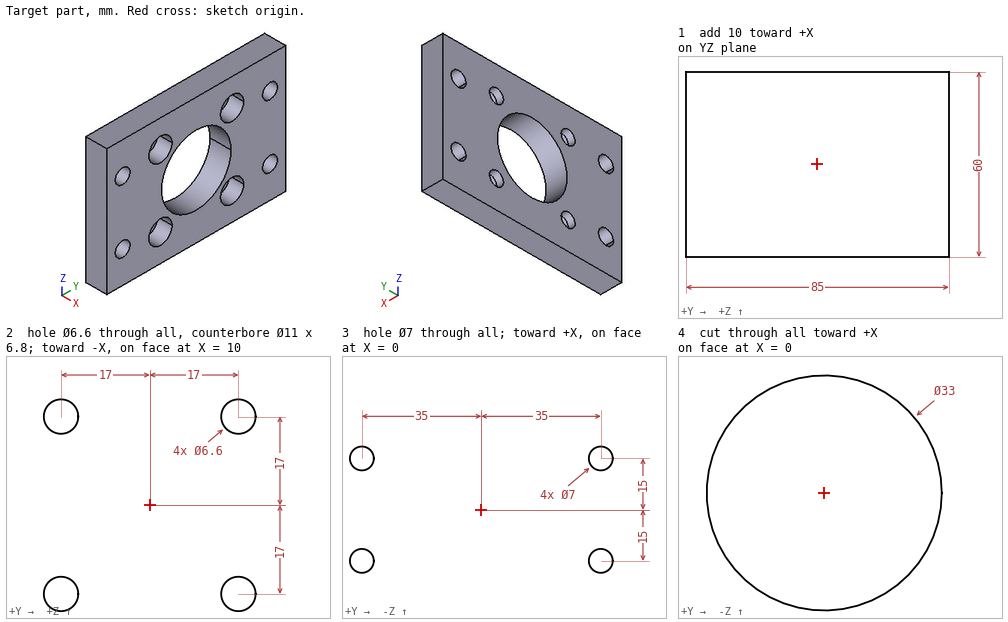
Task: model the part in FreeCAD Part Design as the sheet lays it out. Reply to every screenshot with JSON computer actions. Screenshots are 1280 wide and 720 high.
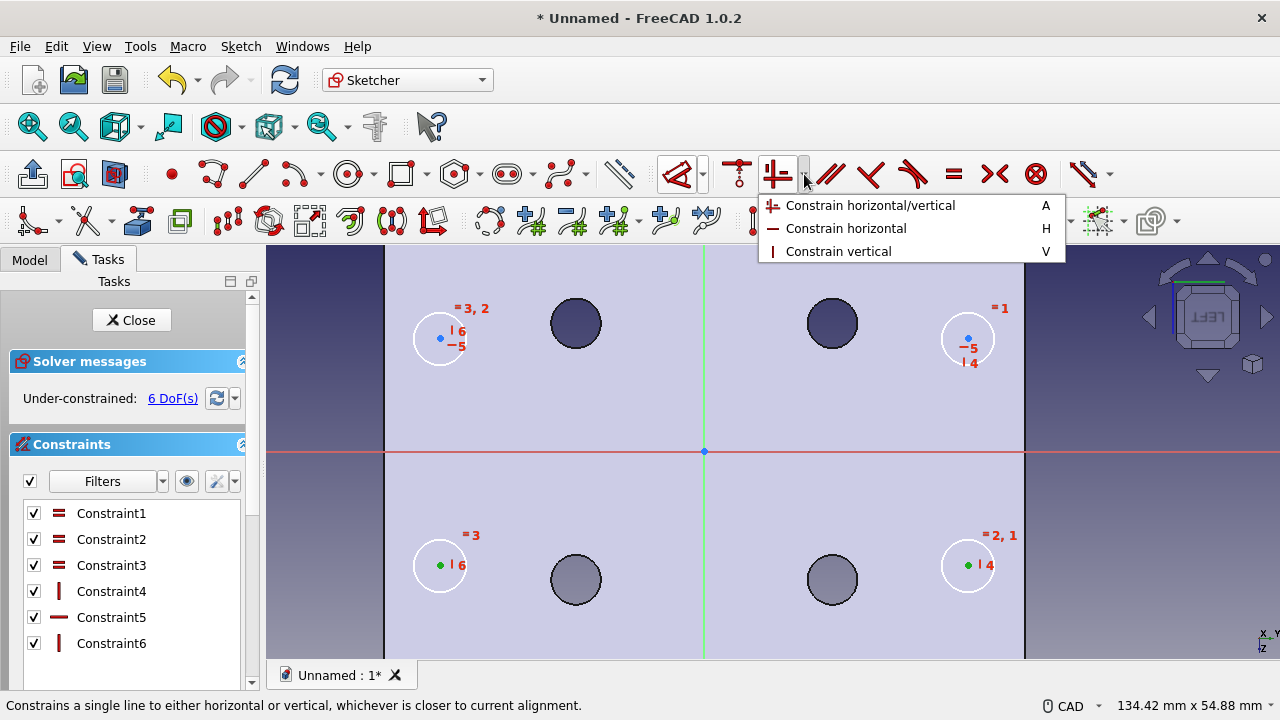
{"action": "left_click", "coordinate": [912, 228]}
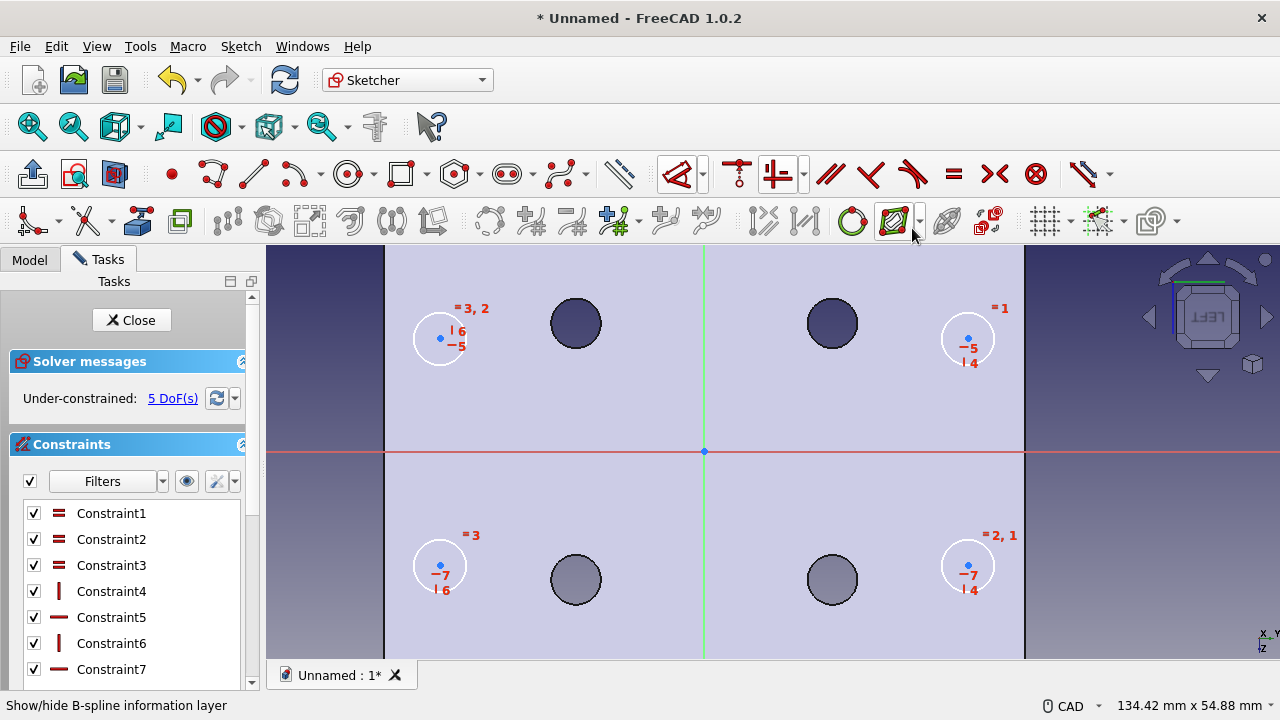
{"action": "left_click", "coordinate": [986, 320]}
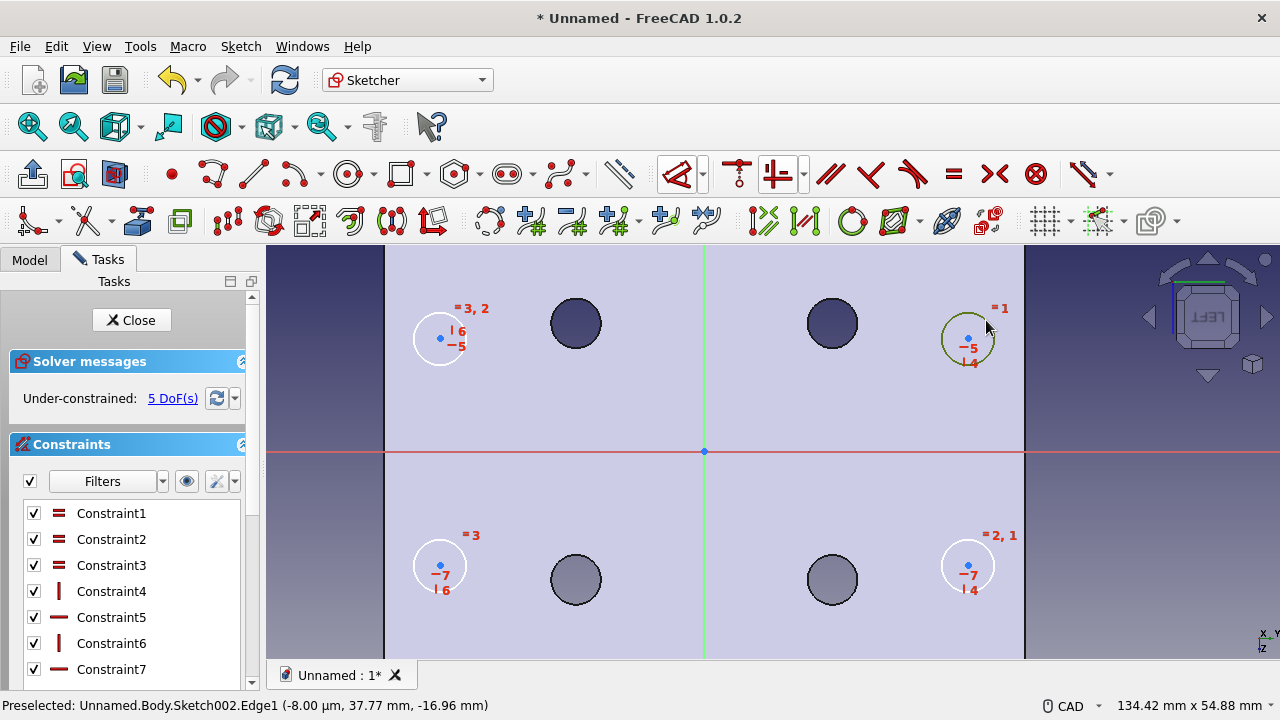
{"action": "key", "text": "k o"}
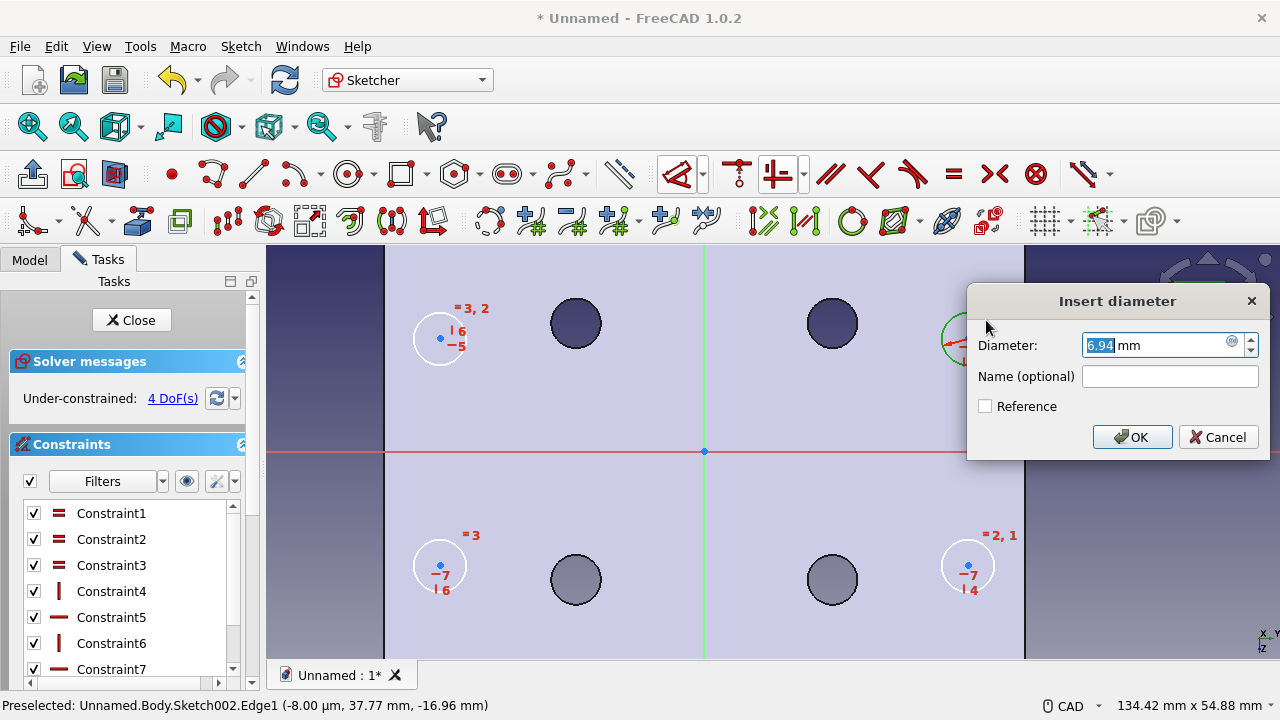
{"action": "type", "text": "7"}
{"action": "key", "text": "Return"}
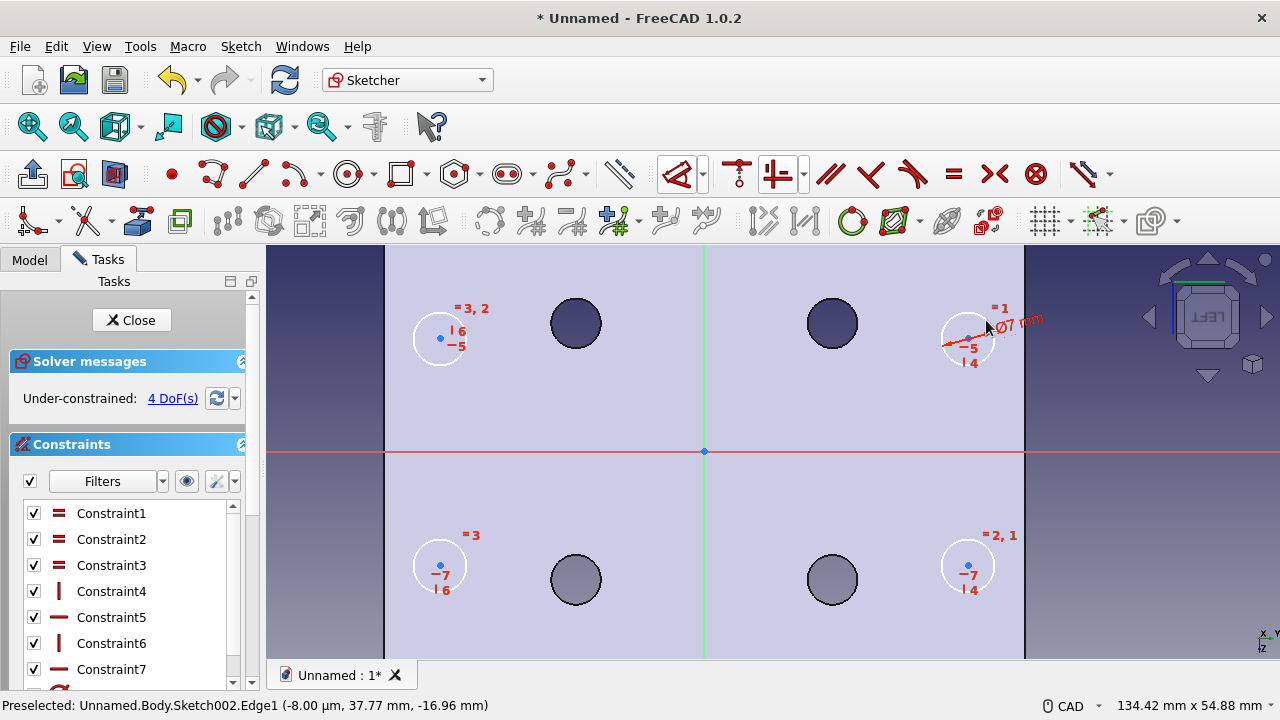
{"action": "left_click", "coordinate": [968, 339]}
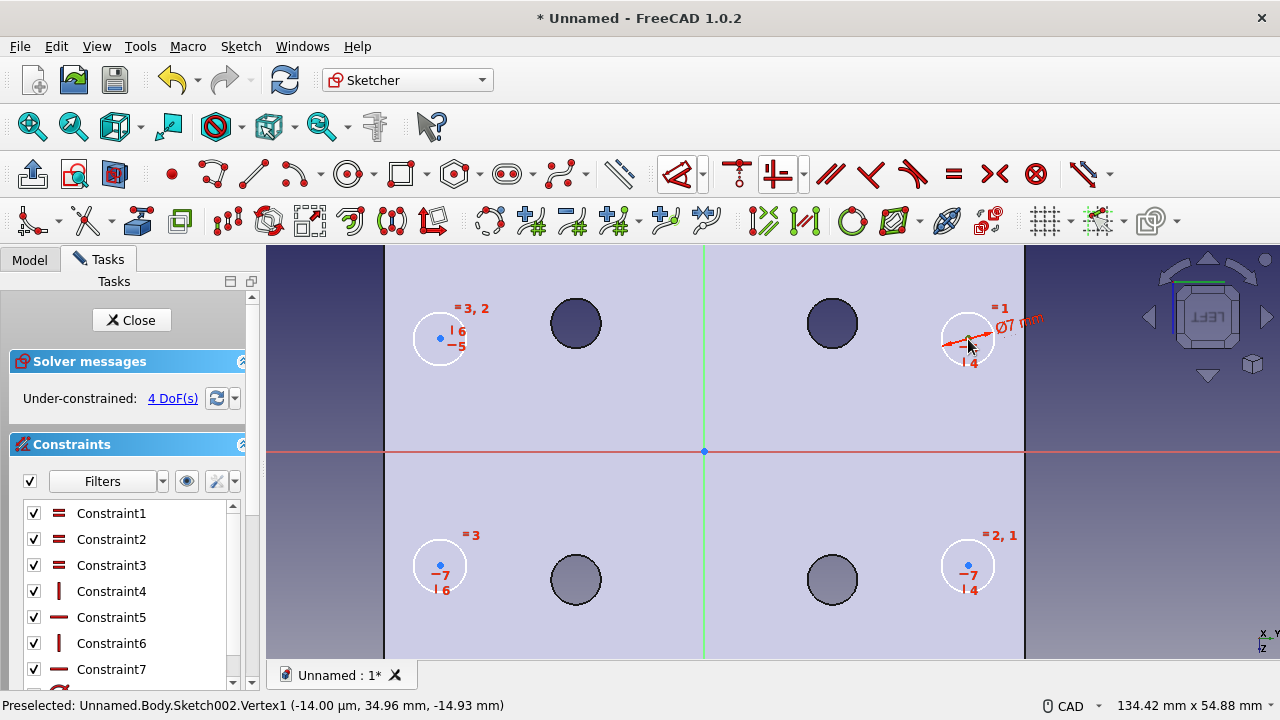
{"action": "key", "text": "l"}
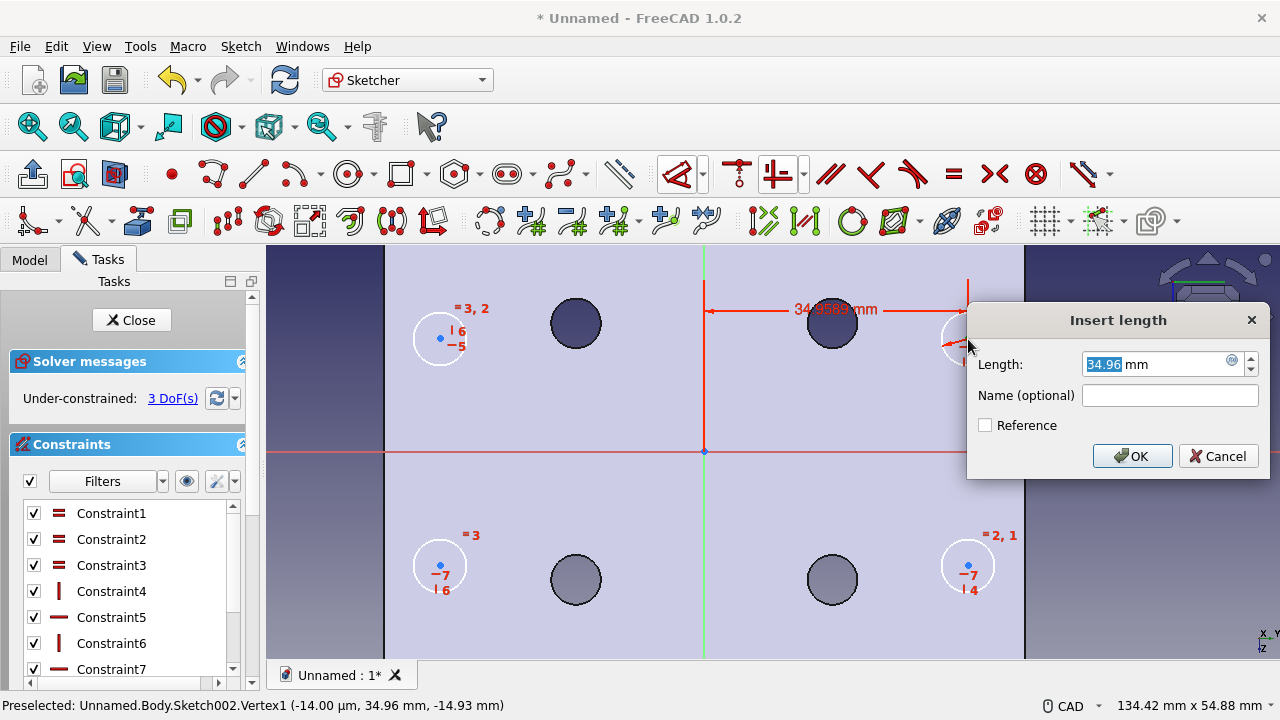
{"action": "type", "text": "35"}
{"action": "key", "text": "Return"}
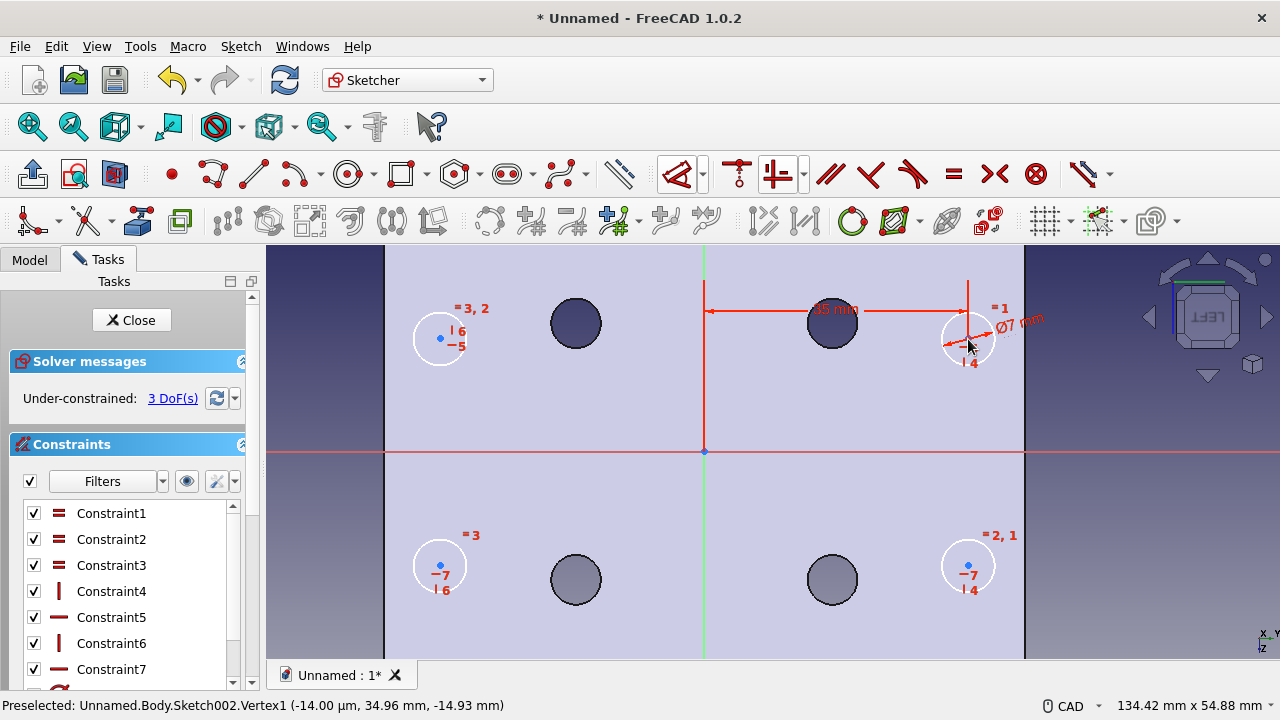
{"action": "left_click", "coordinate": [968, 339]}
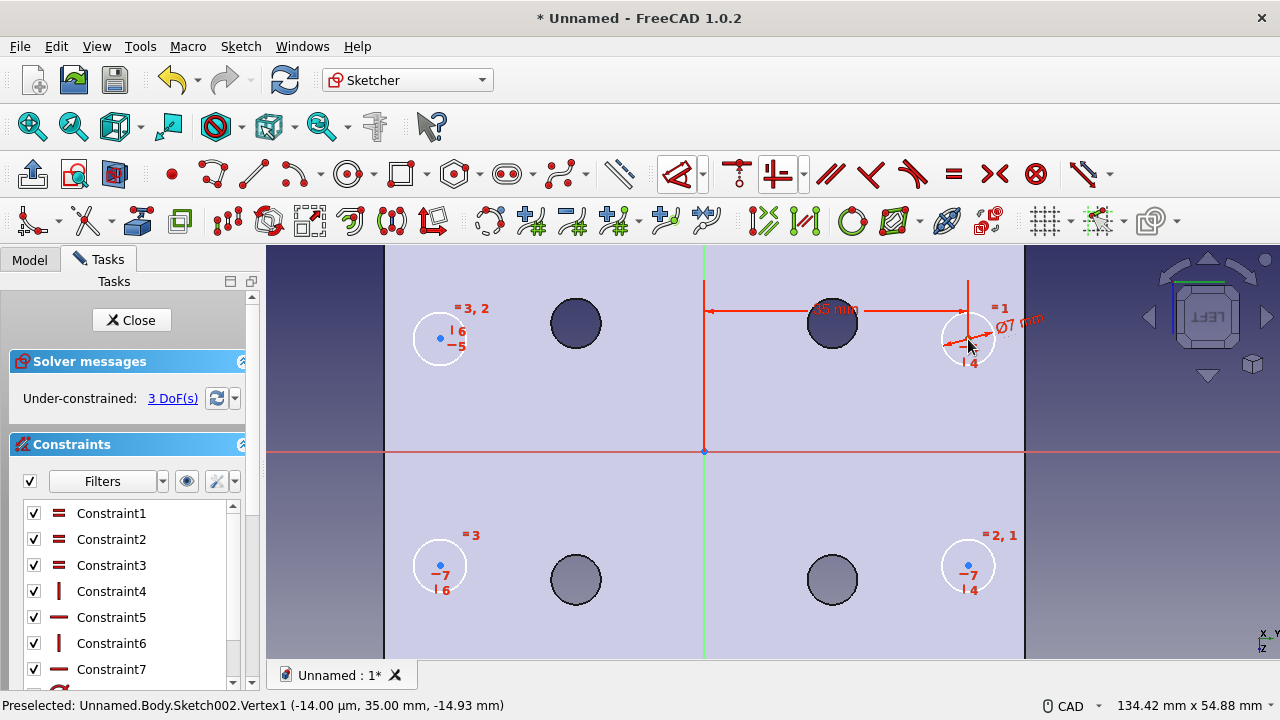
{"action": "key", "text": "i"}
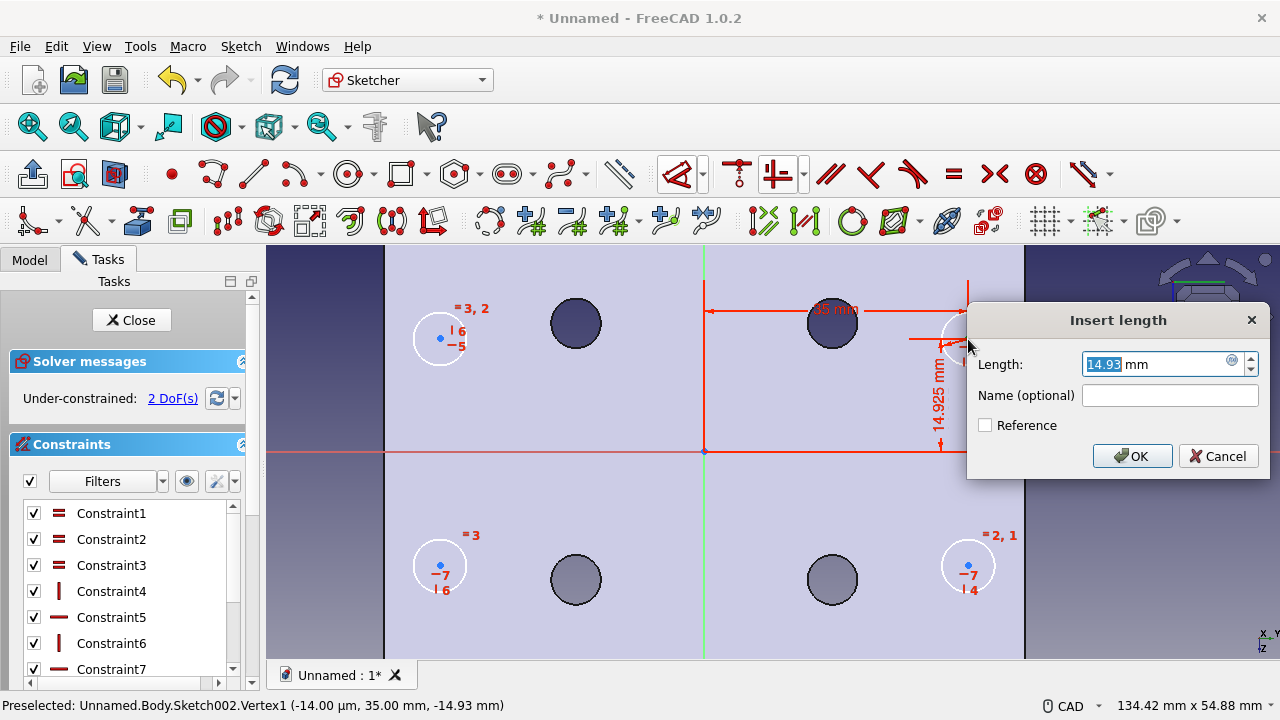
{"action": "type", "text": "15"}
{"action": "key", "text": "Return"}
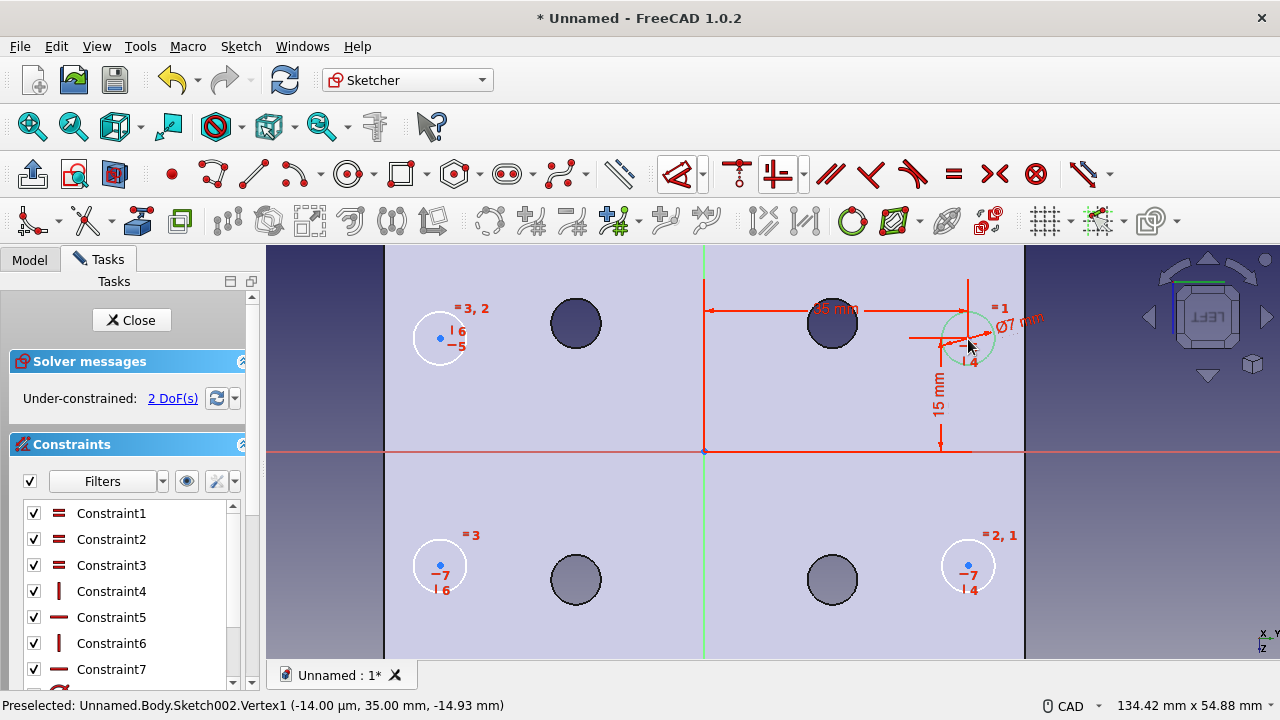
{"action": "left_click", "coordinate": [968, 566]}